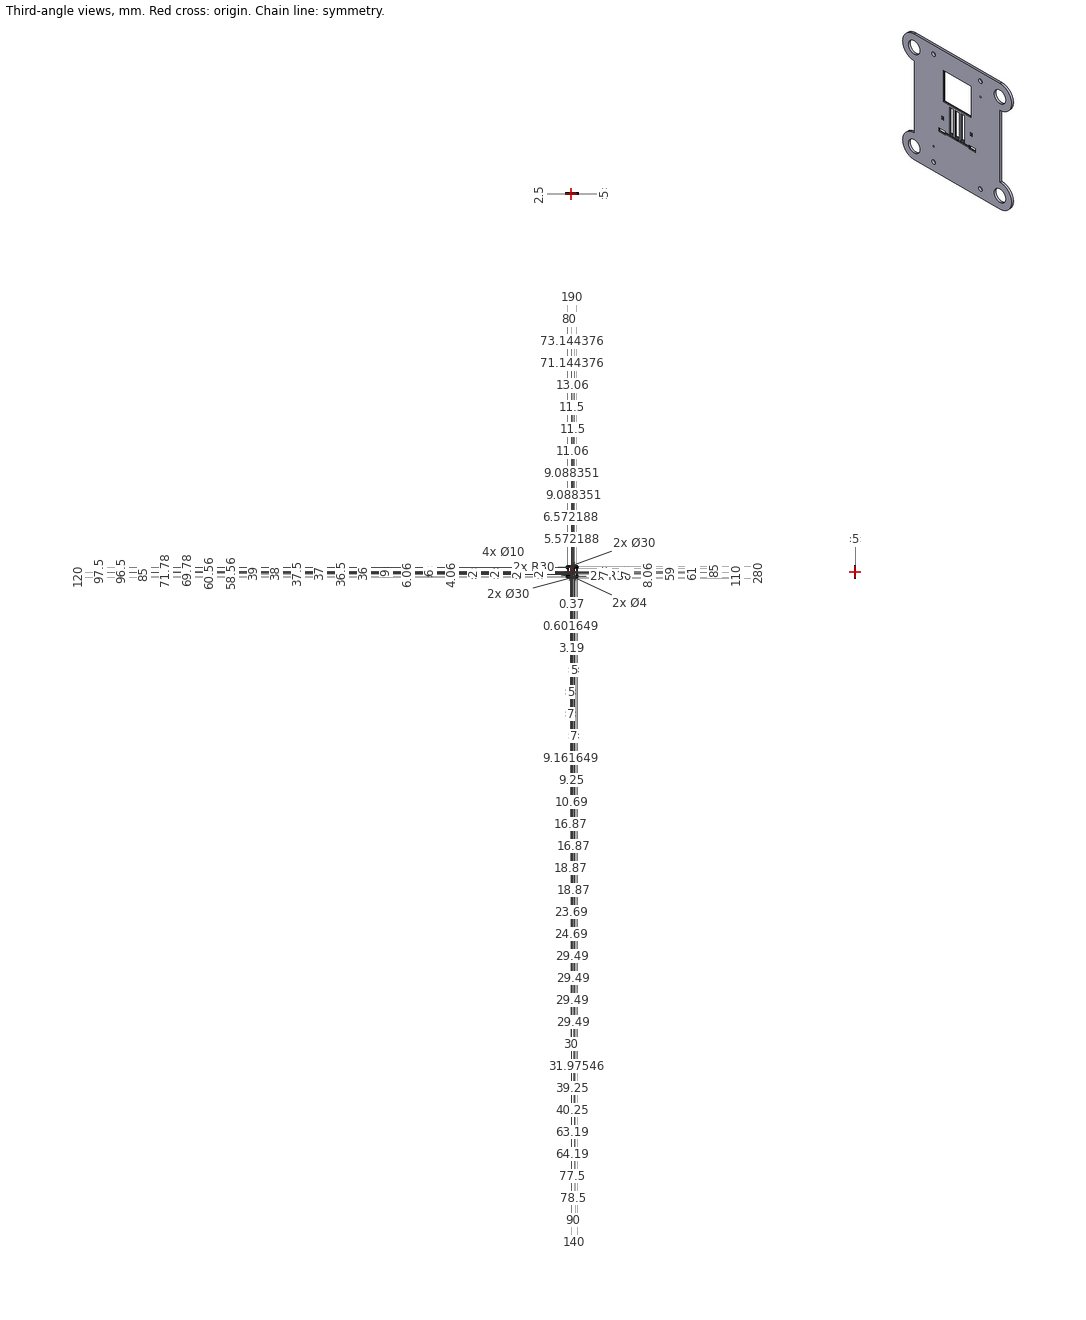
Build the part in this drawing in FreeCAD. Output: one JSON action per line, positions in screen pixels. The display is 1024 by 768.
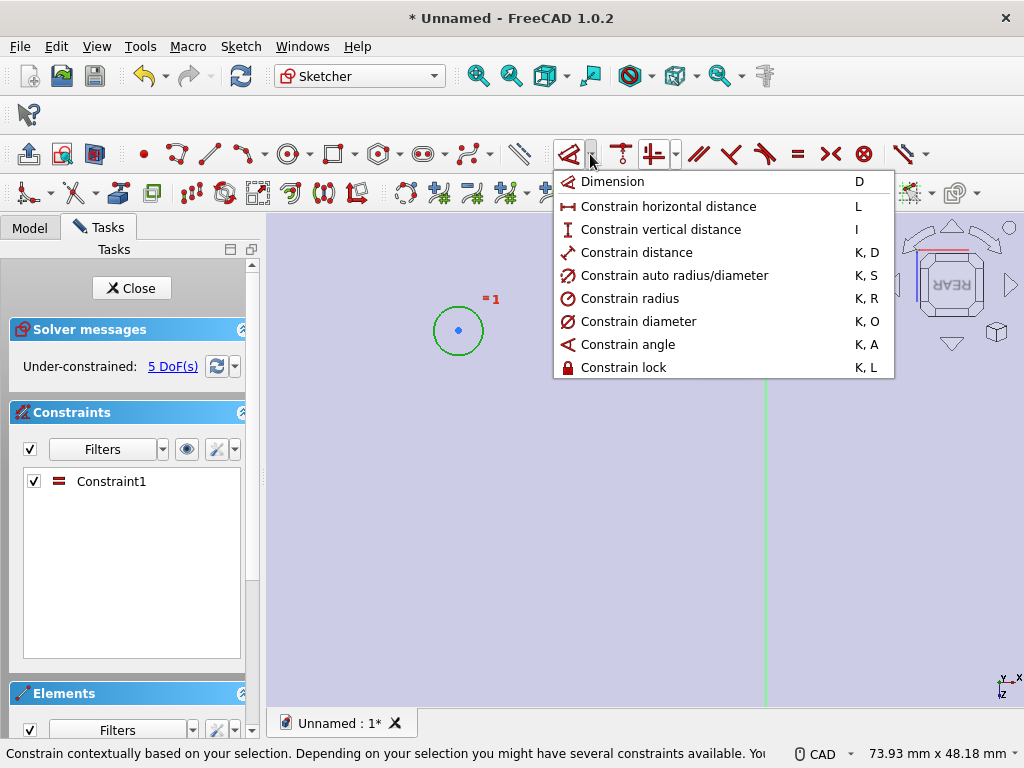
{"action": "left_click", "coordinate": [724, 322]}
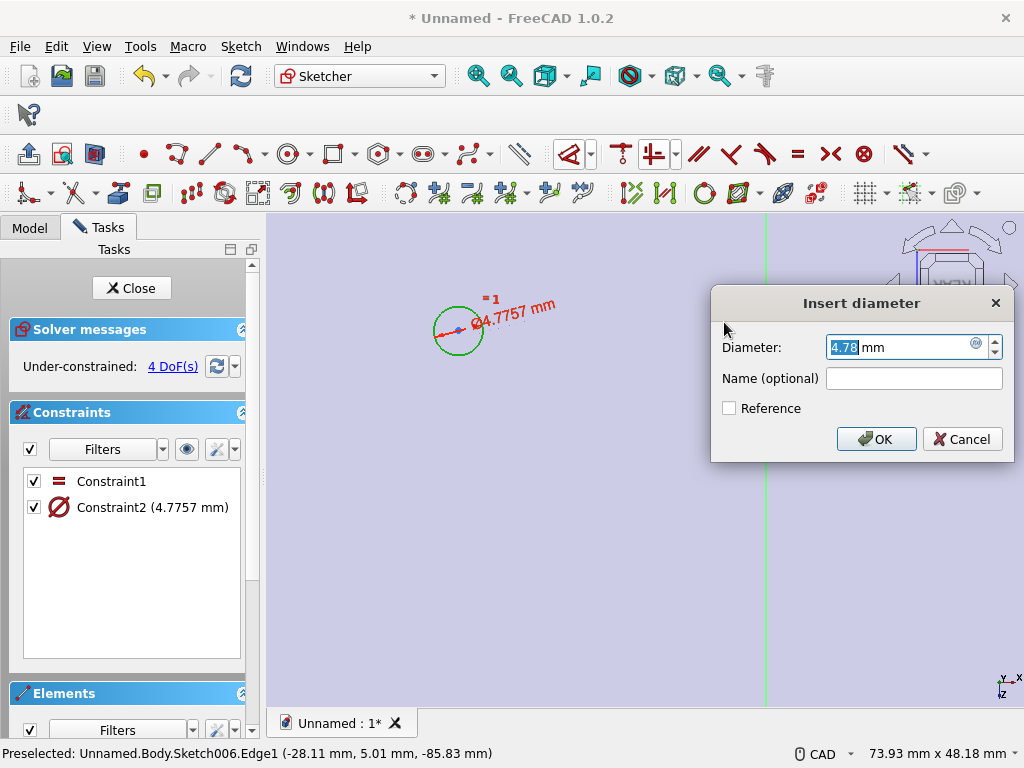
{"action": "type", "text": "4"}
{"action": "key", "text": "Return"}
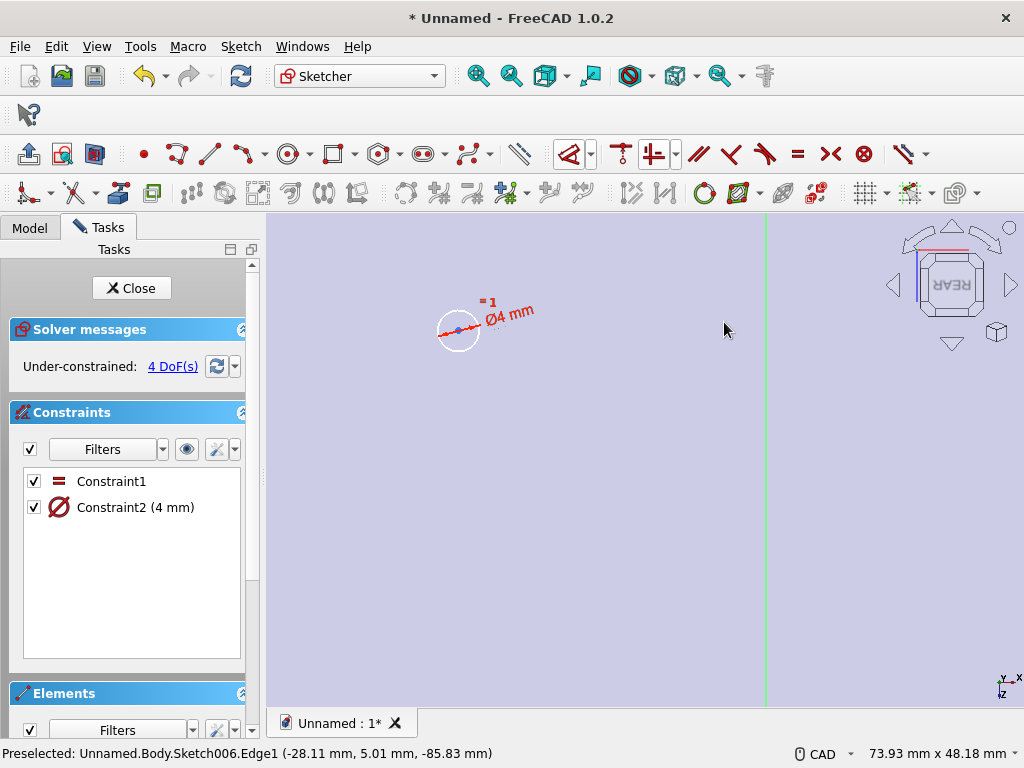
{"action": "scroll", "coordinate": [478, 314], "scroll_direction": "down", "scroll_amount": 9}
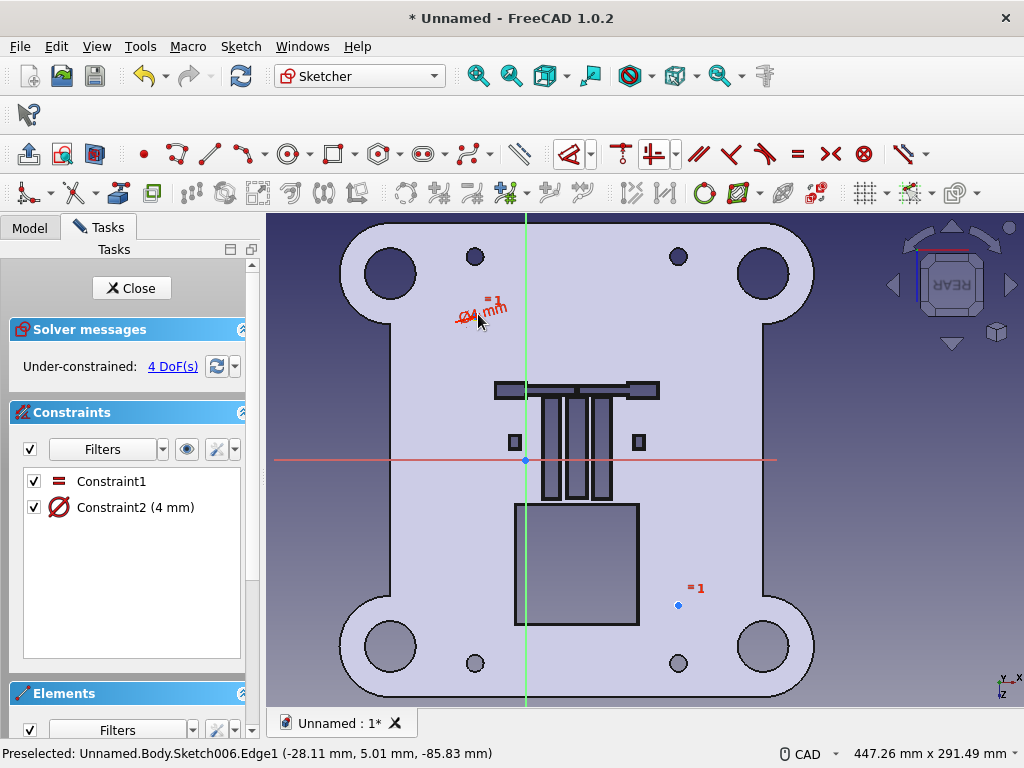
{"action": "left_click", "coordinate": [475, 317]}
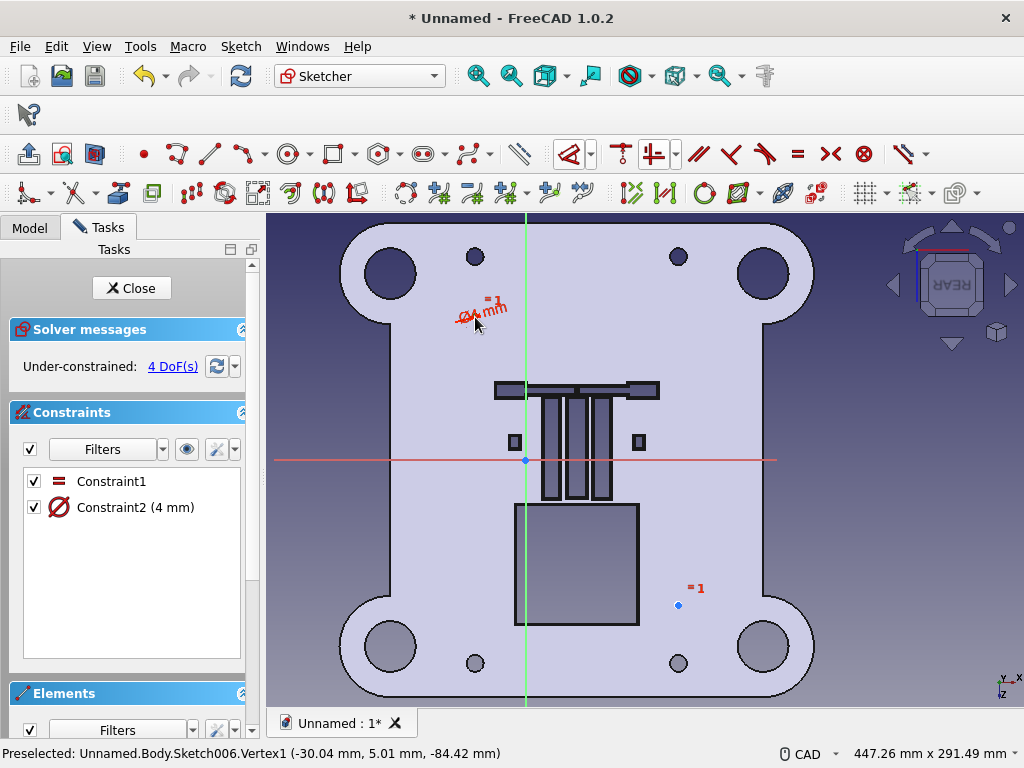
{"action": "key", "text": "l"}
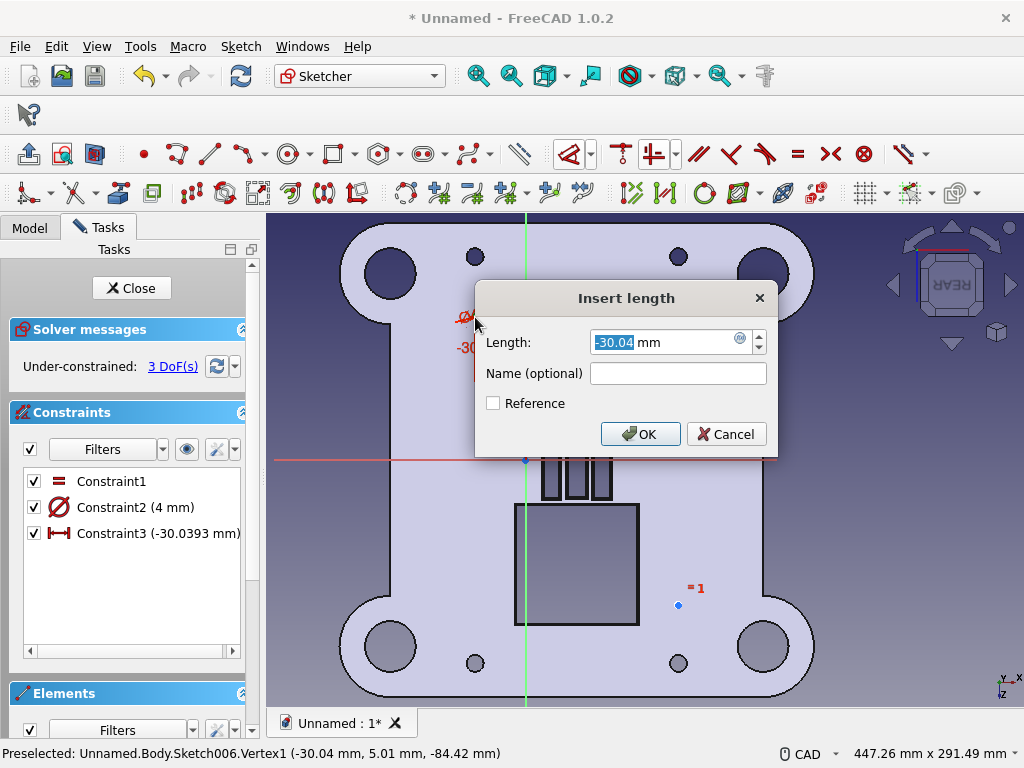
{"action": "type", "text": "-30"}
{"action": "key", "text": "Return"}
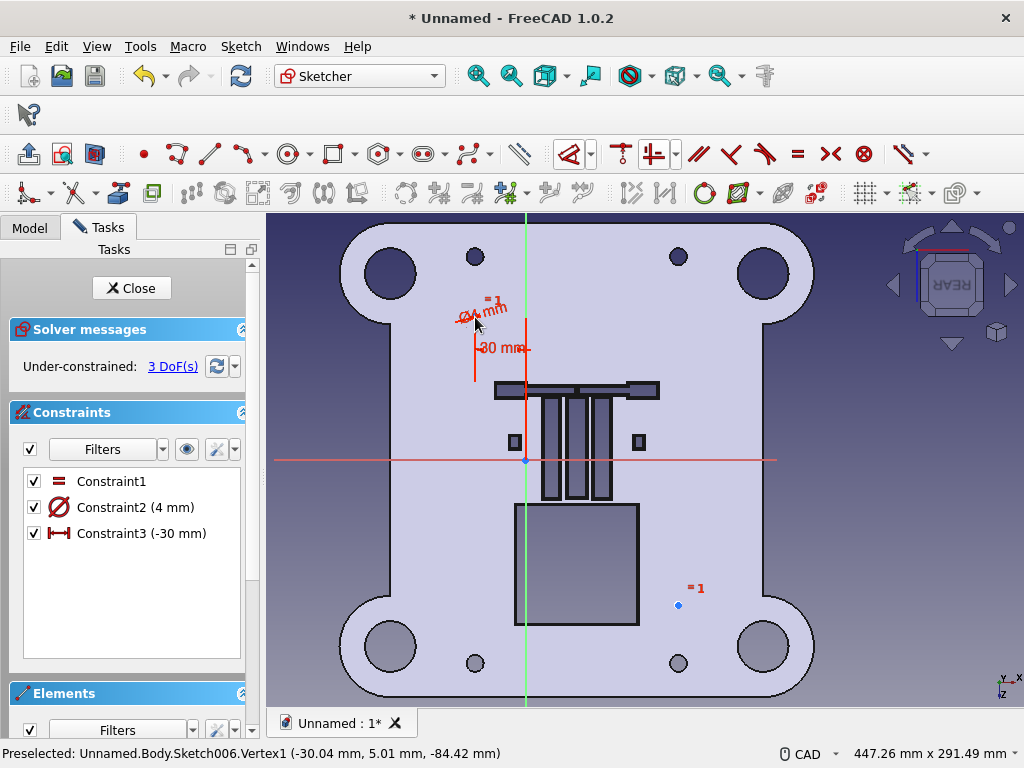
{"action": "left_click", "coordinate": [475, 317]}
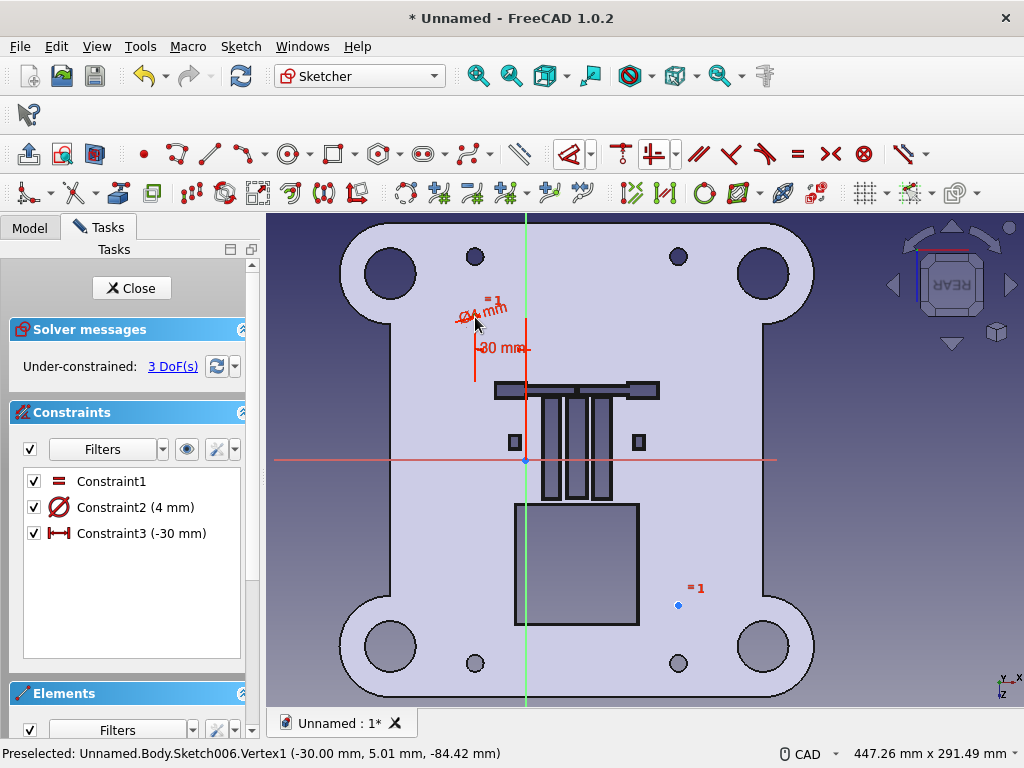
{"action": "key", "text": "i"}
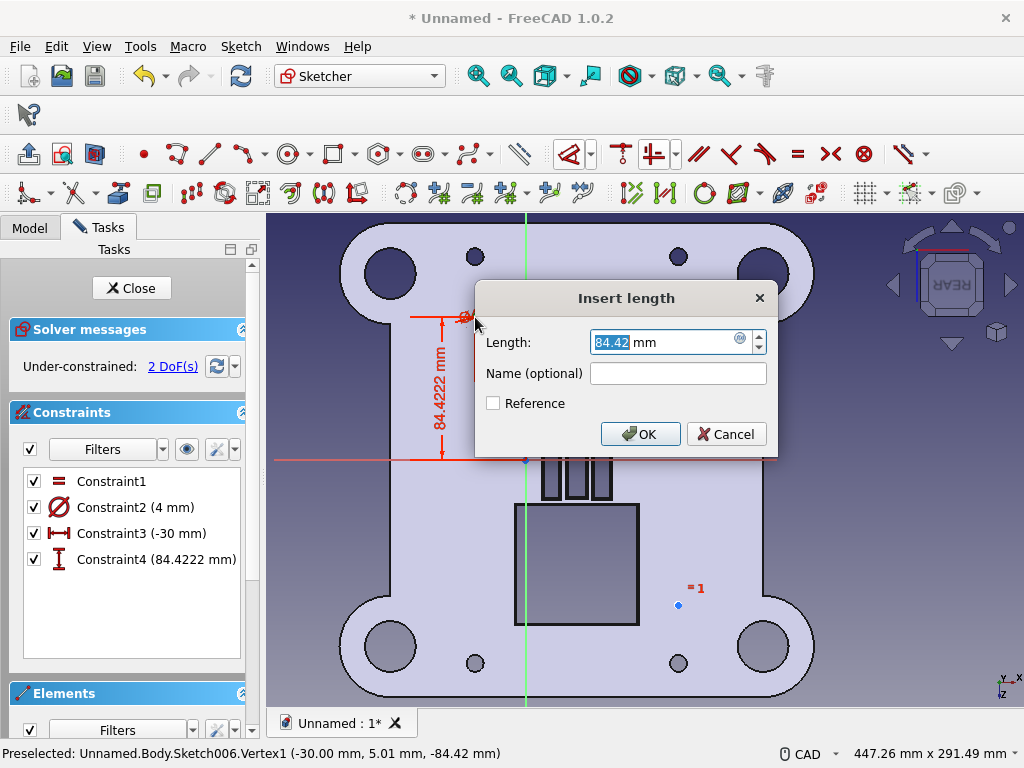
{"action": "type", "text": "85"}
{"action": "key", "text": "Return"}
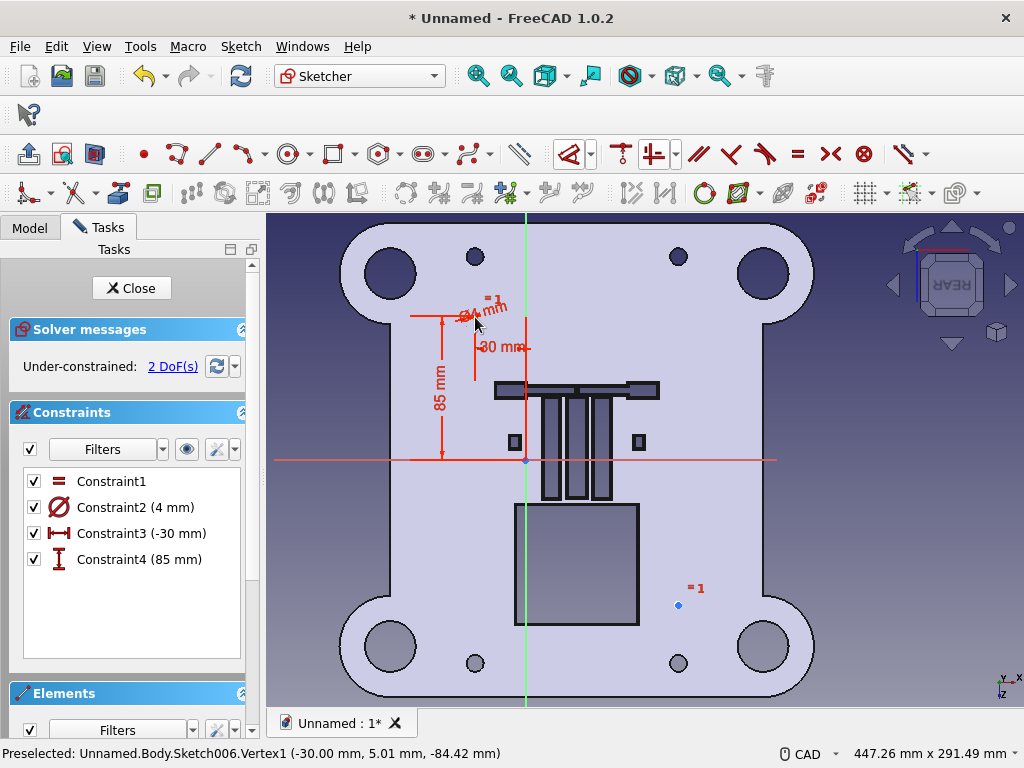
{"action": "left_click", "coordinate": [678, 605]}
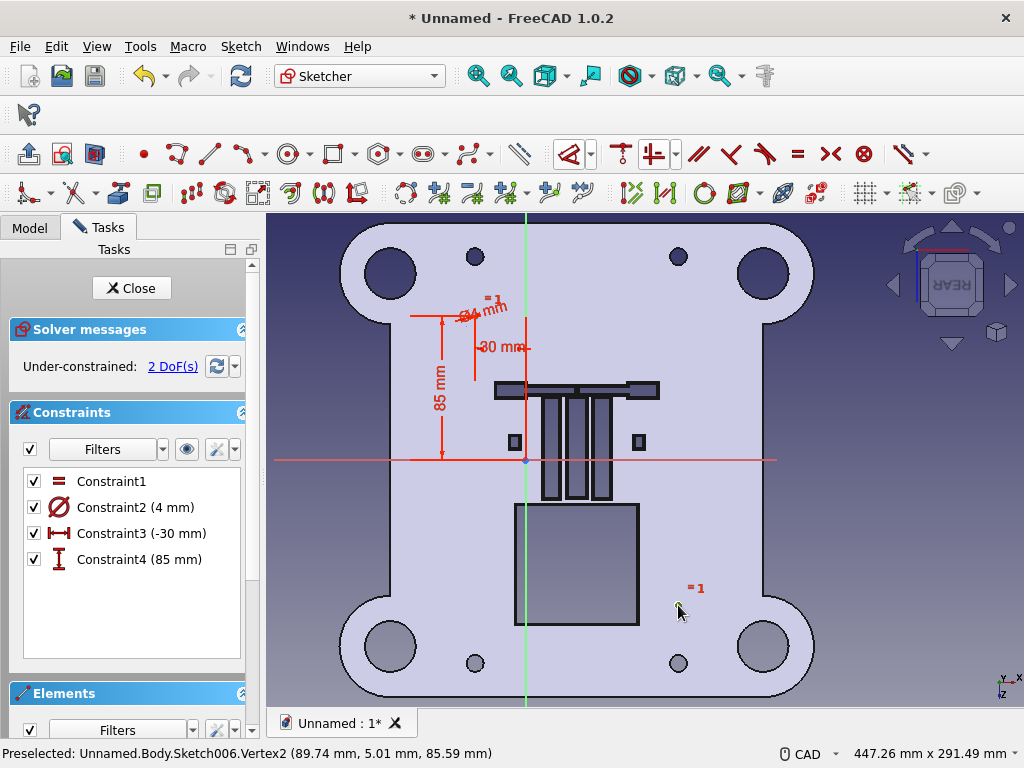
{"action": "key", "text": "l"}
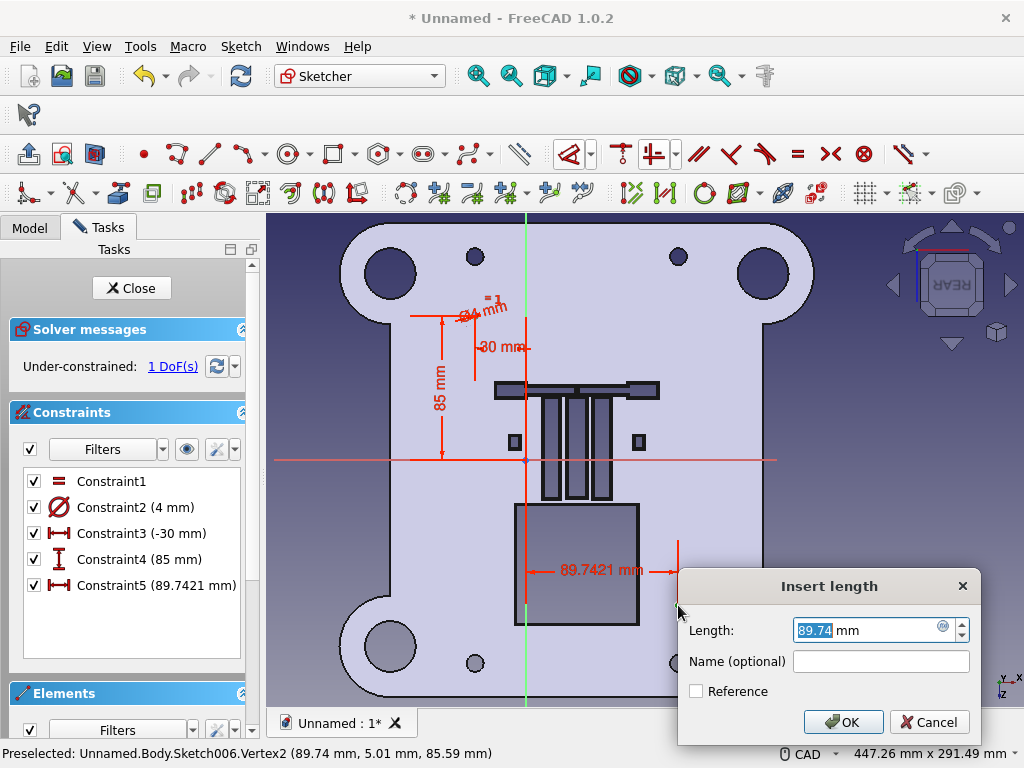
{"action": "type", "text": "90"}
{"action": "key", "text": "Return"}